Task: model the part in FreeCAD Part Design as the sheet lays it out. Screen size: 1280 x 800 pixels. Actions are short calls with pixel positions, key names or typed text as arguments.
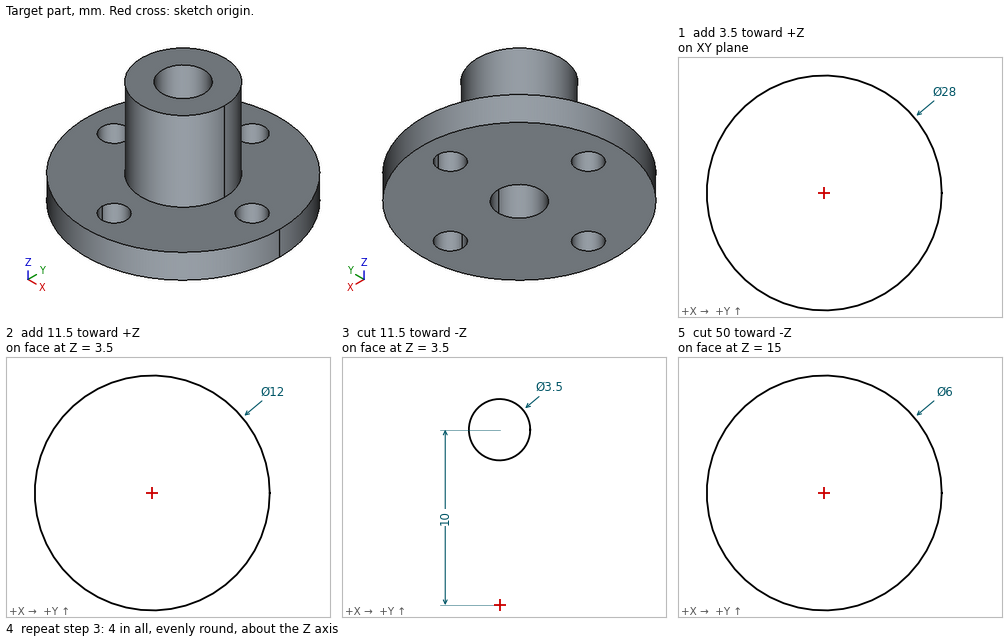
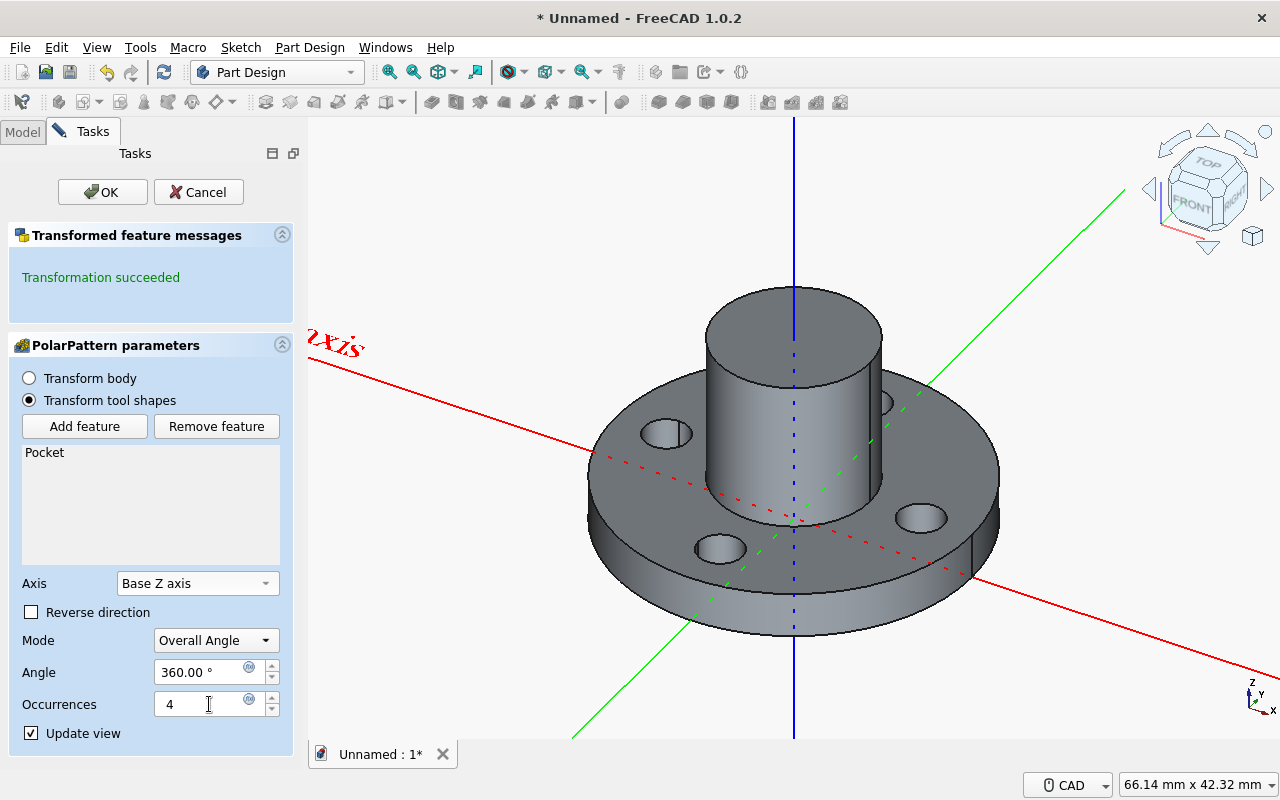
click(103, 192)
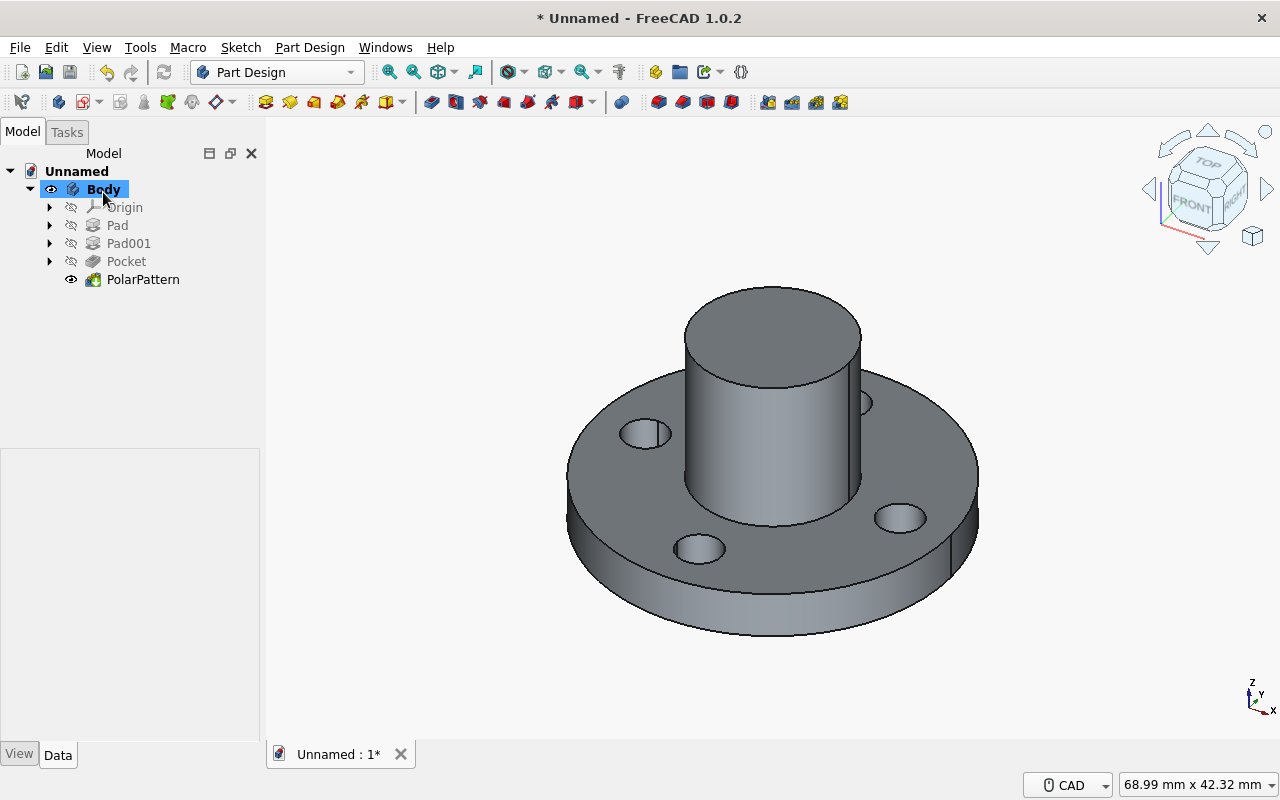
click(773, 337)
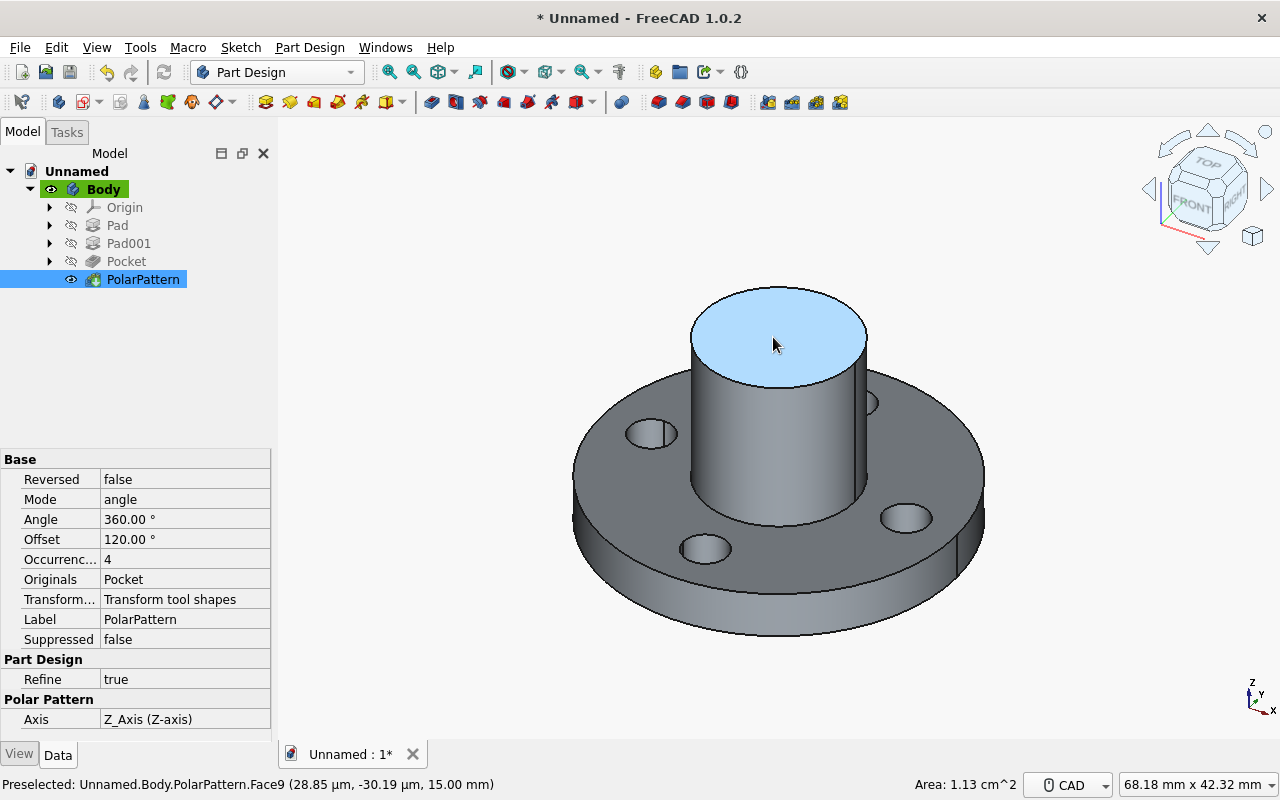
click(84, 102)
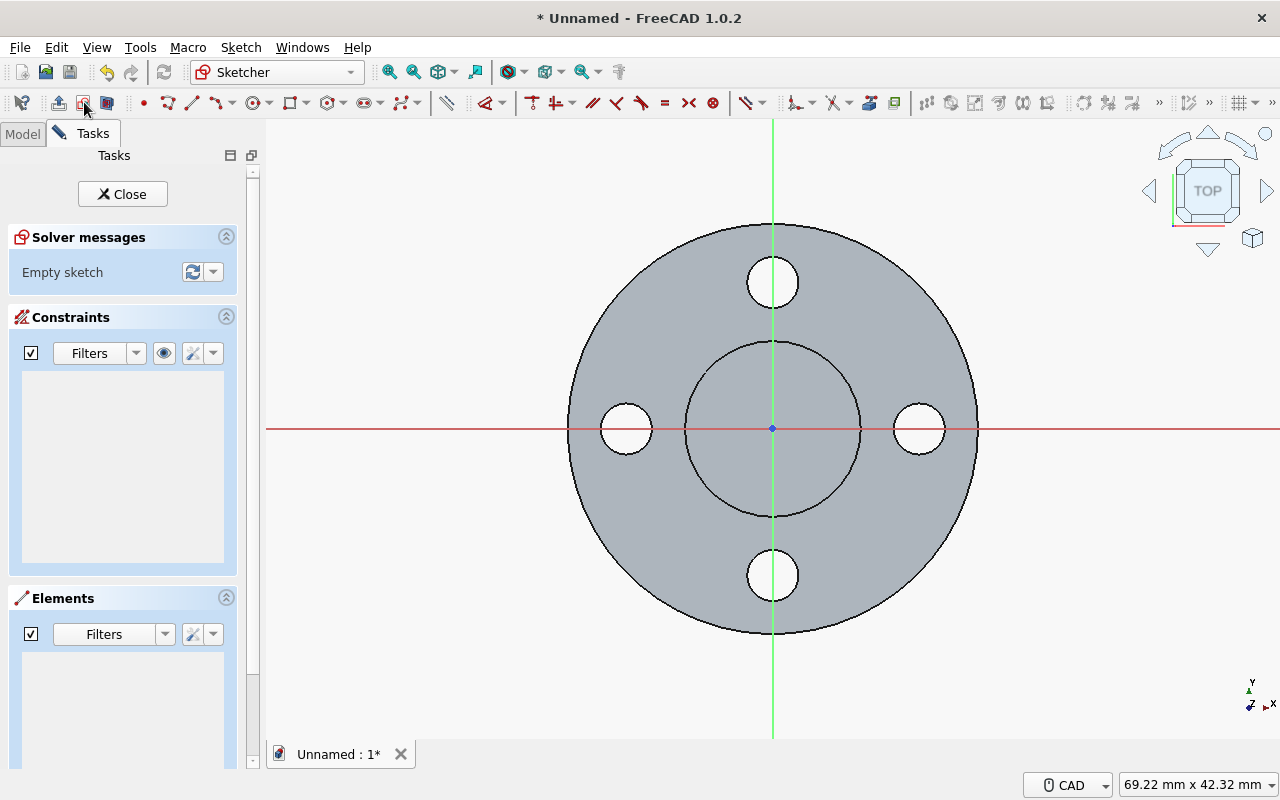
scroll(790, 429, up, 8)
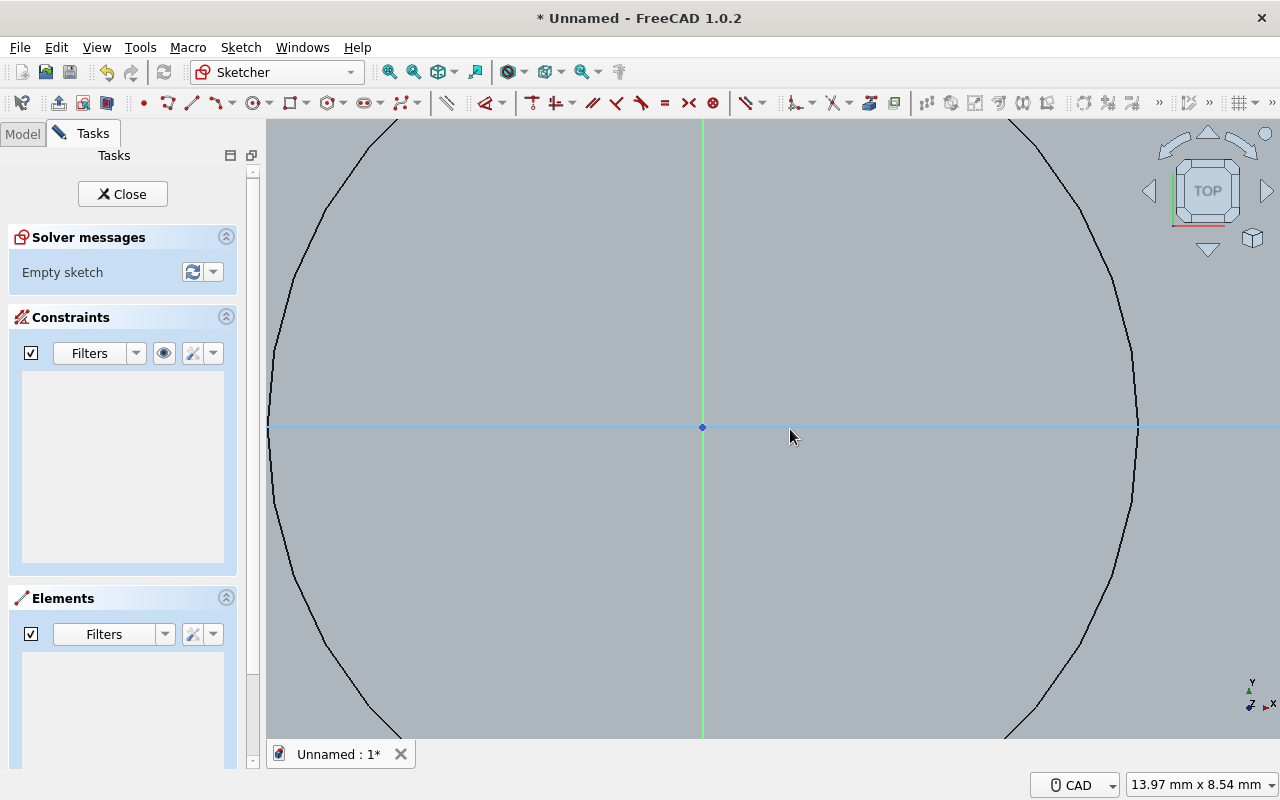
click(254, 104)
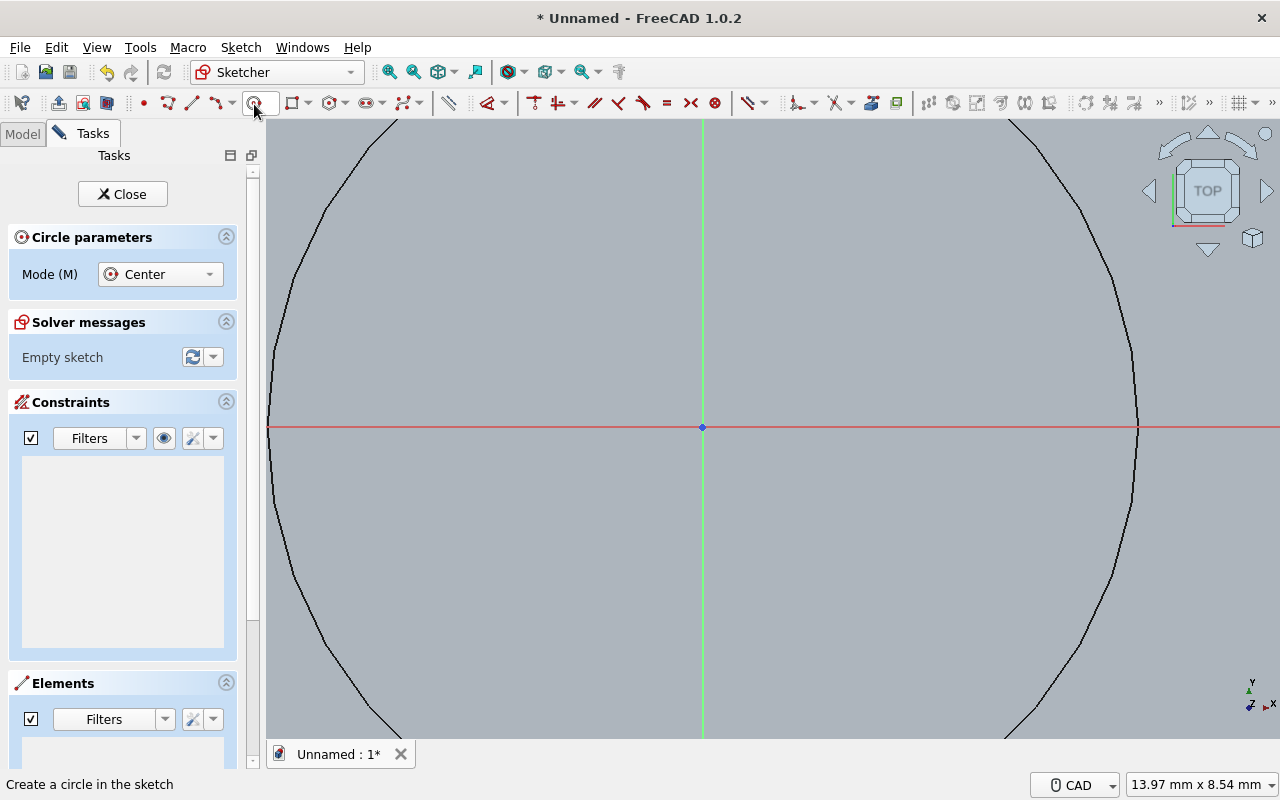
click(703, 427)
click(857, 273)
key(Escape)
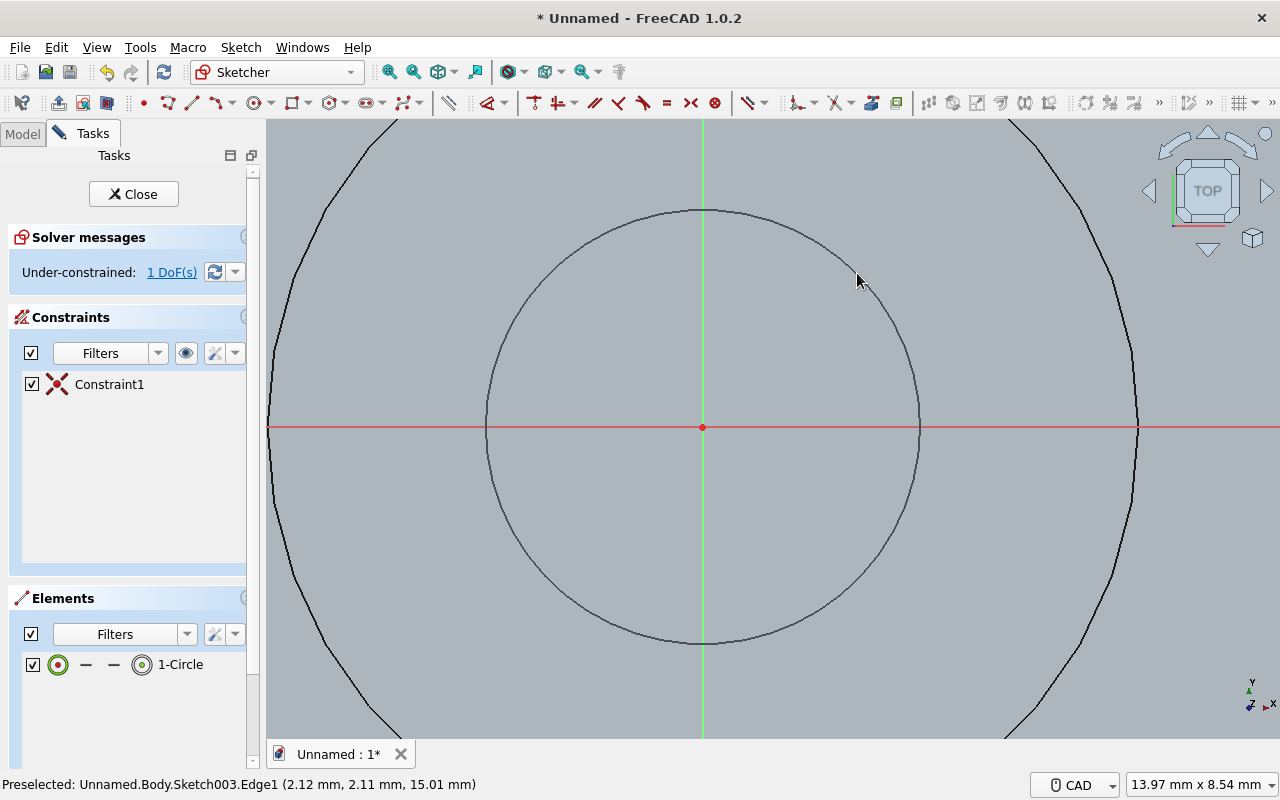
key(d)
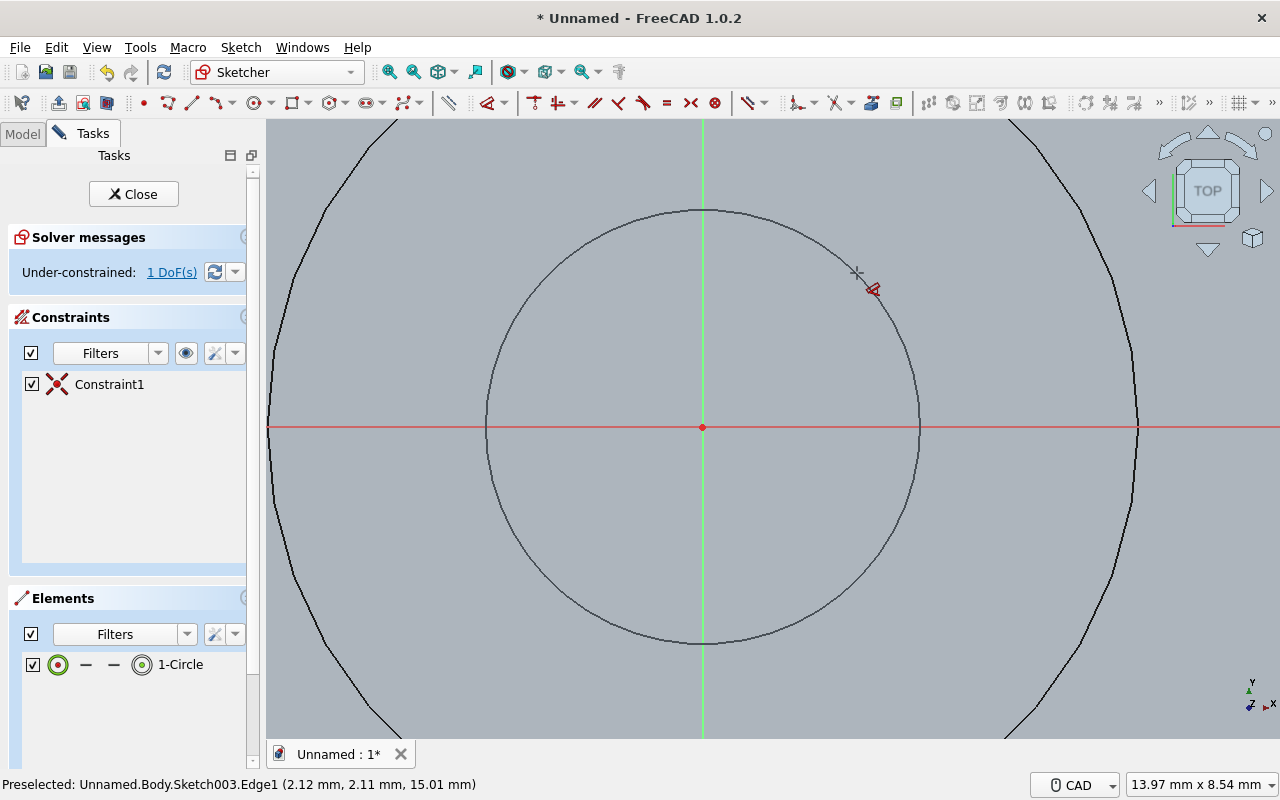
click(856, 273)
click(879, 250)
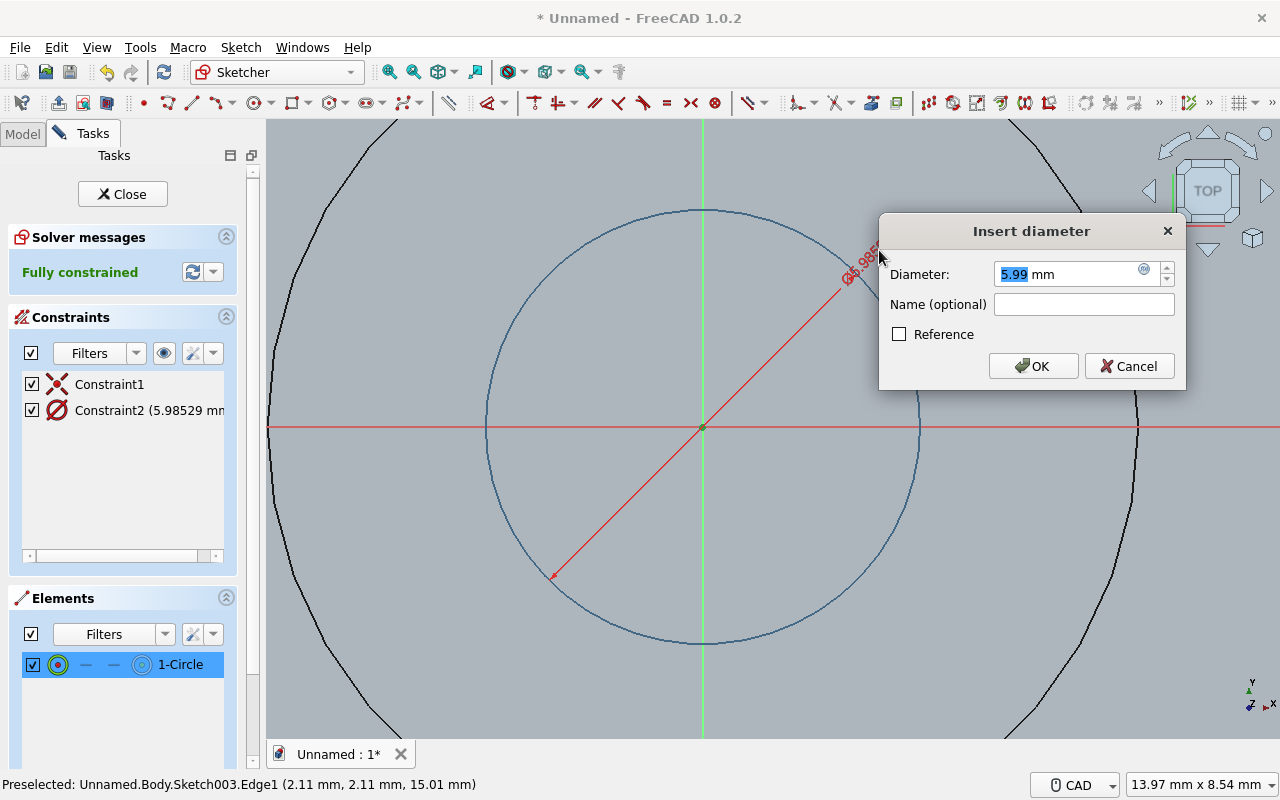
text(6)
key(Return)
key(Escape)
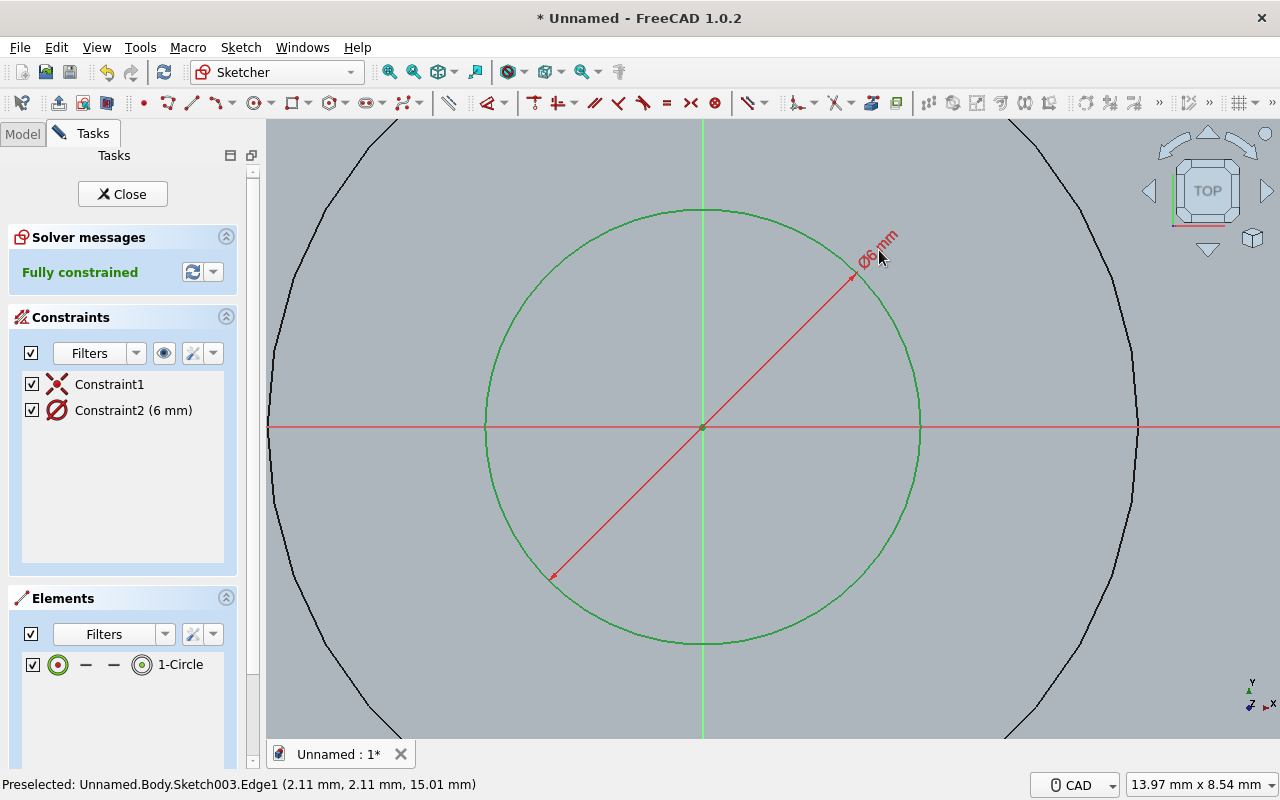
click(123, 194)